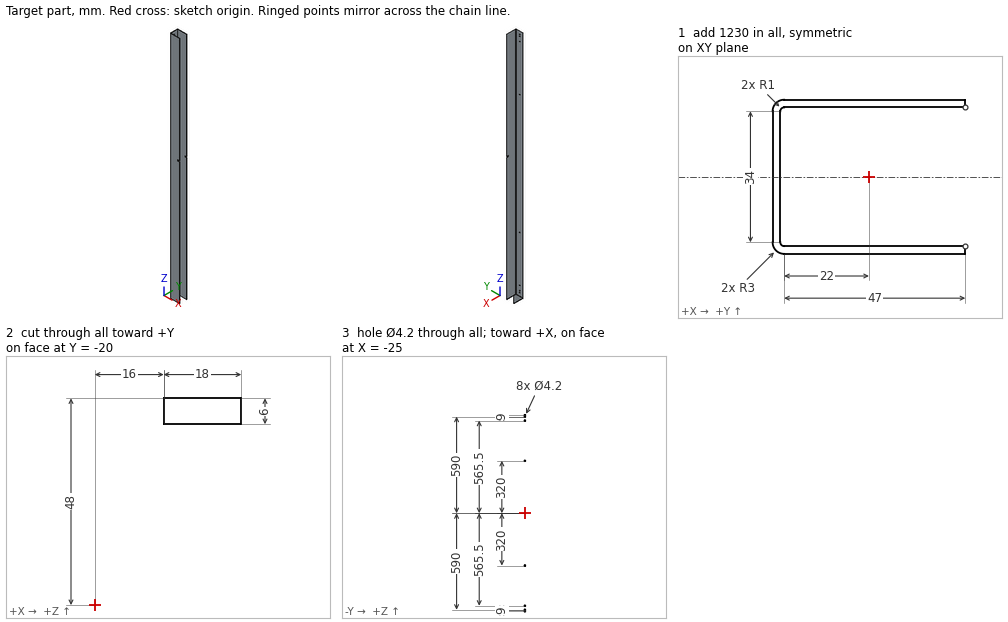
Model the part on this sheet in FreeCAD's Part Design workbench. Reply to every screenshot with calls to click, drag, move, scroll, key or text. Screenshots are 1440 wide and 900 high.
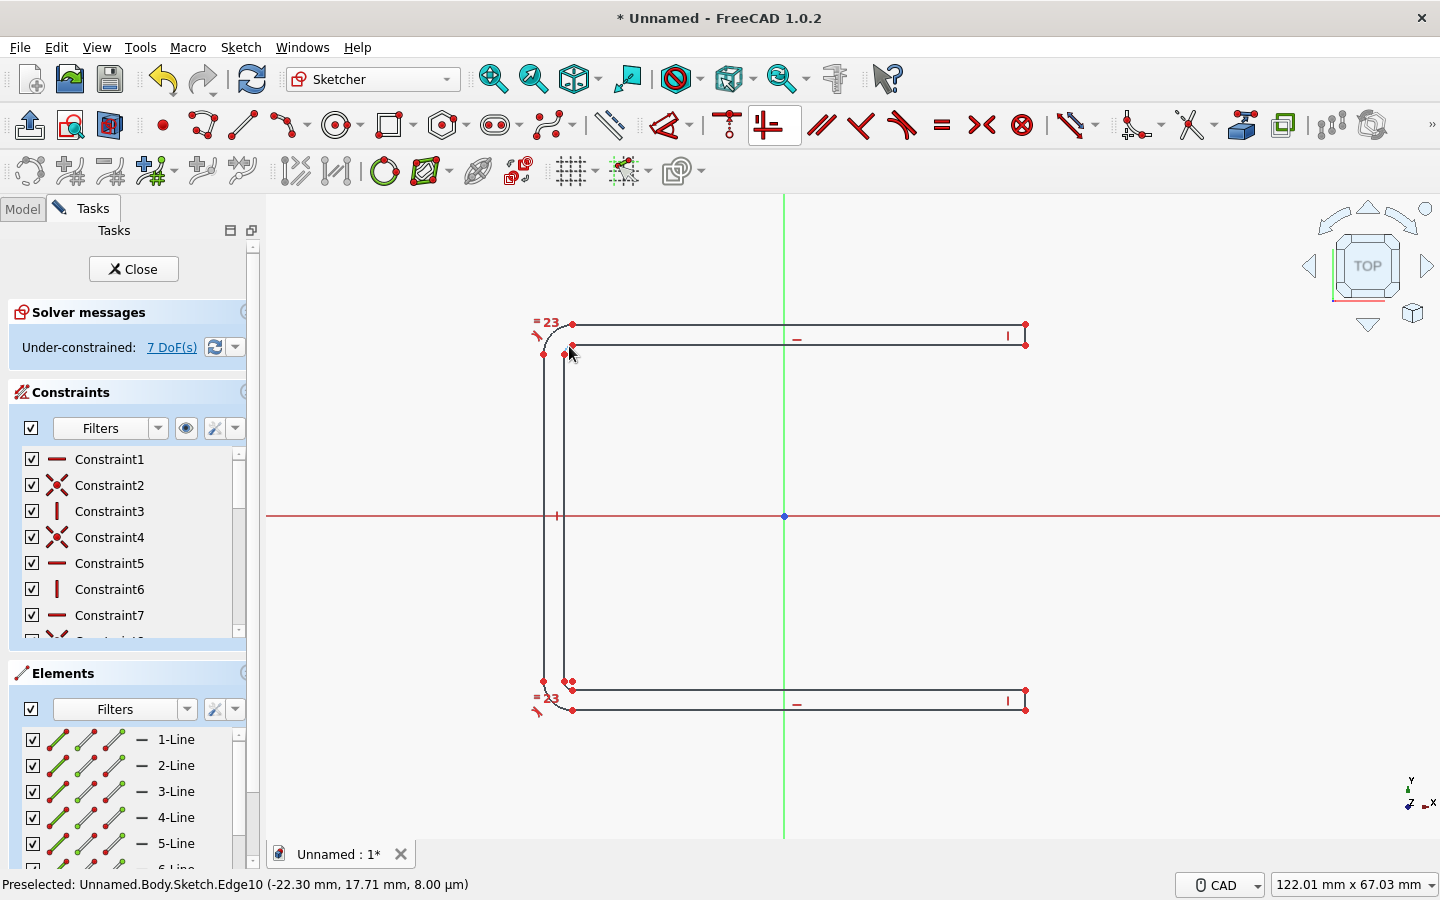
click(1025, 690)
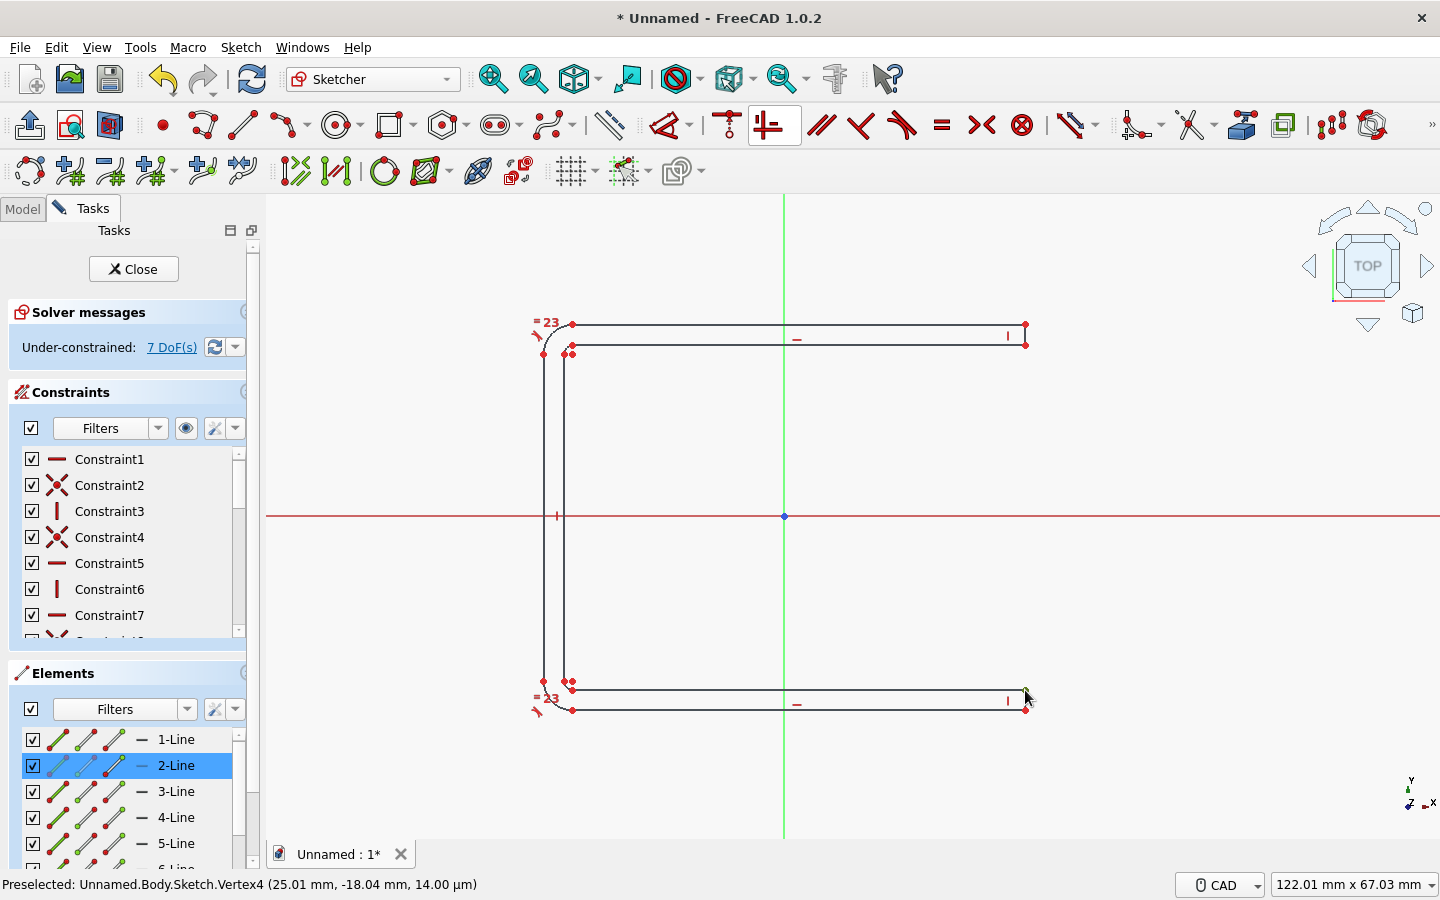
click(1025, 345)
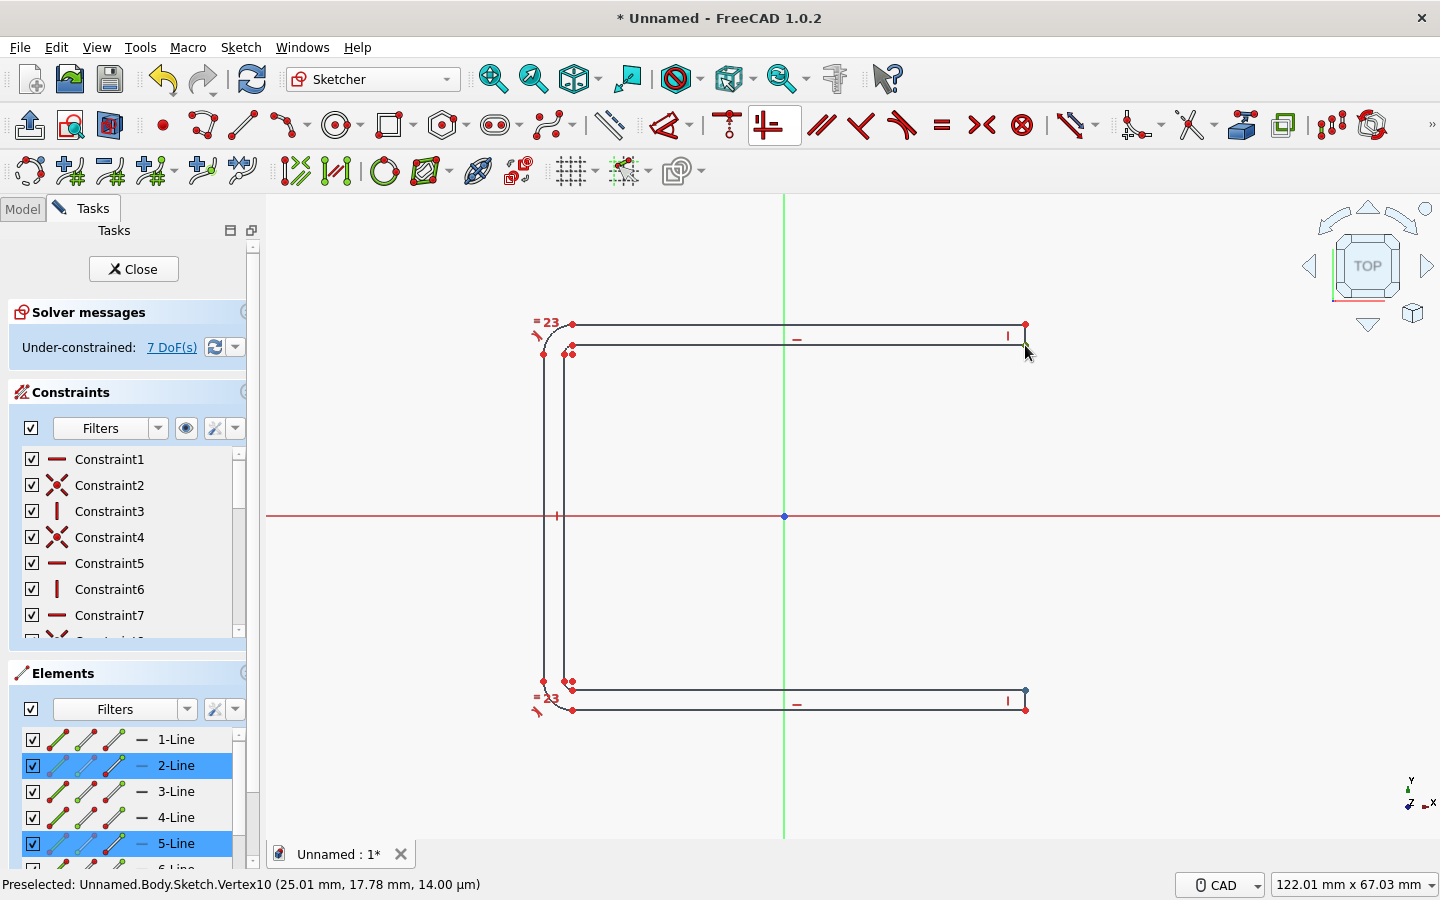
click(364, 516)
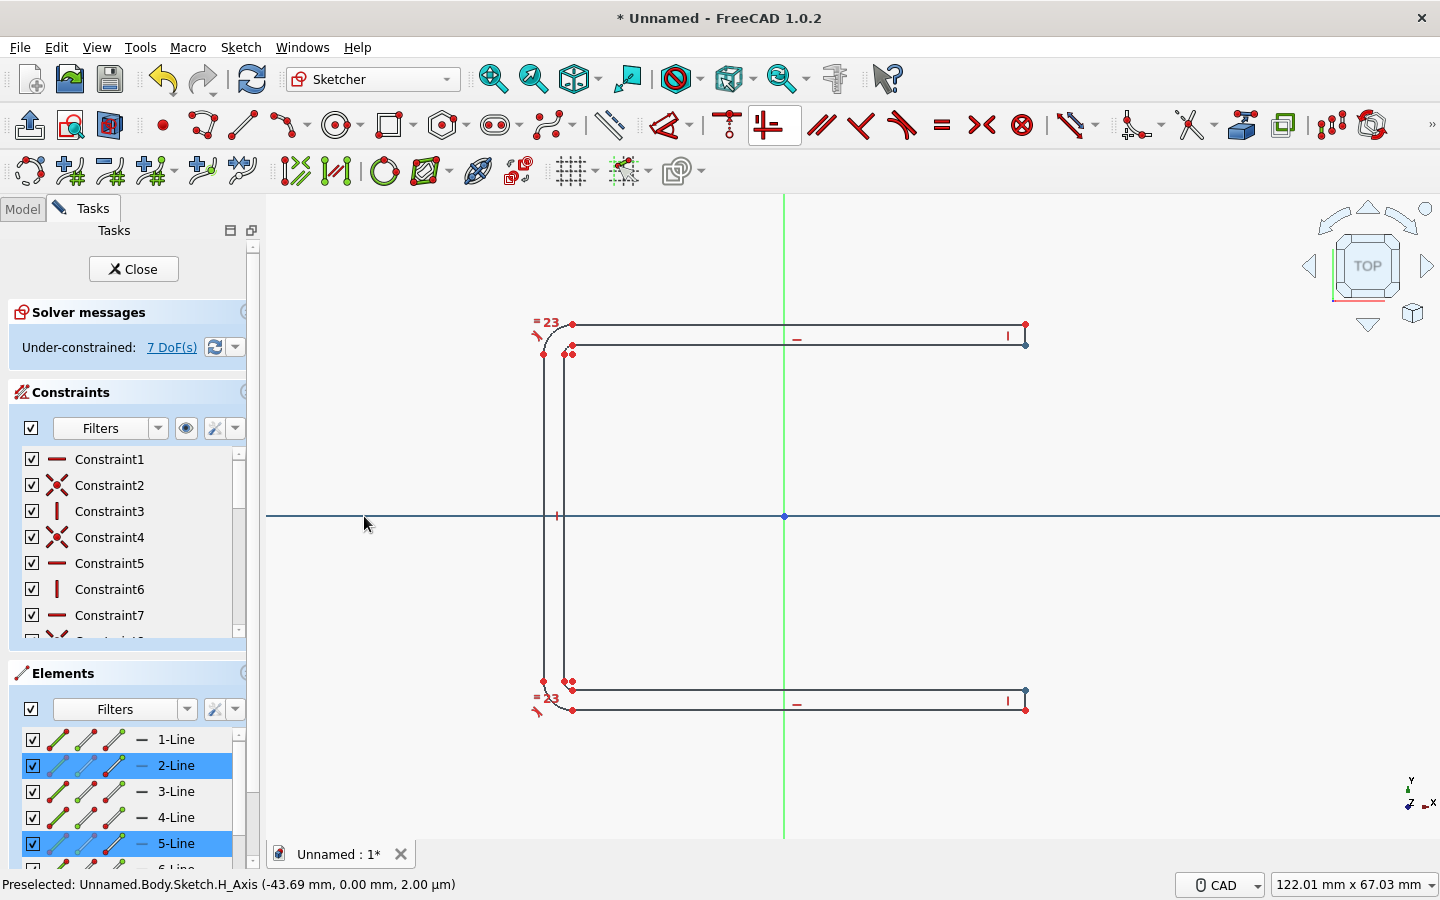
click(982, 126)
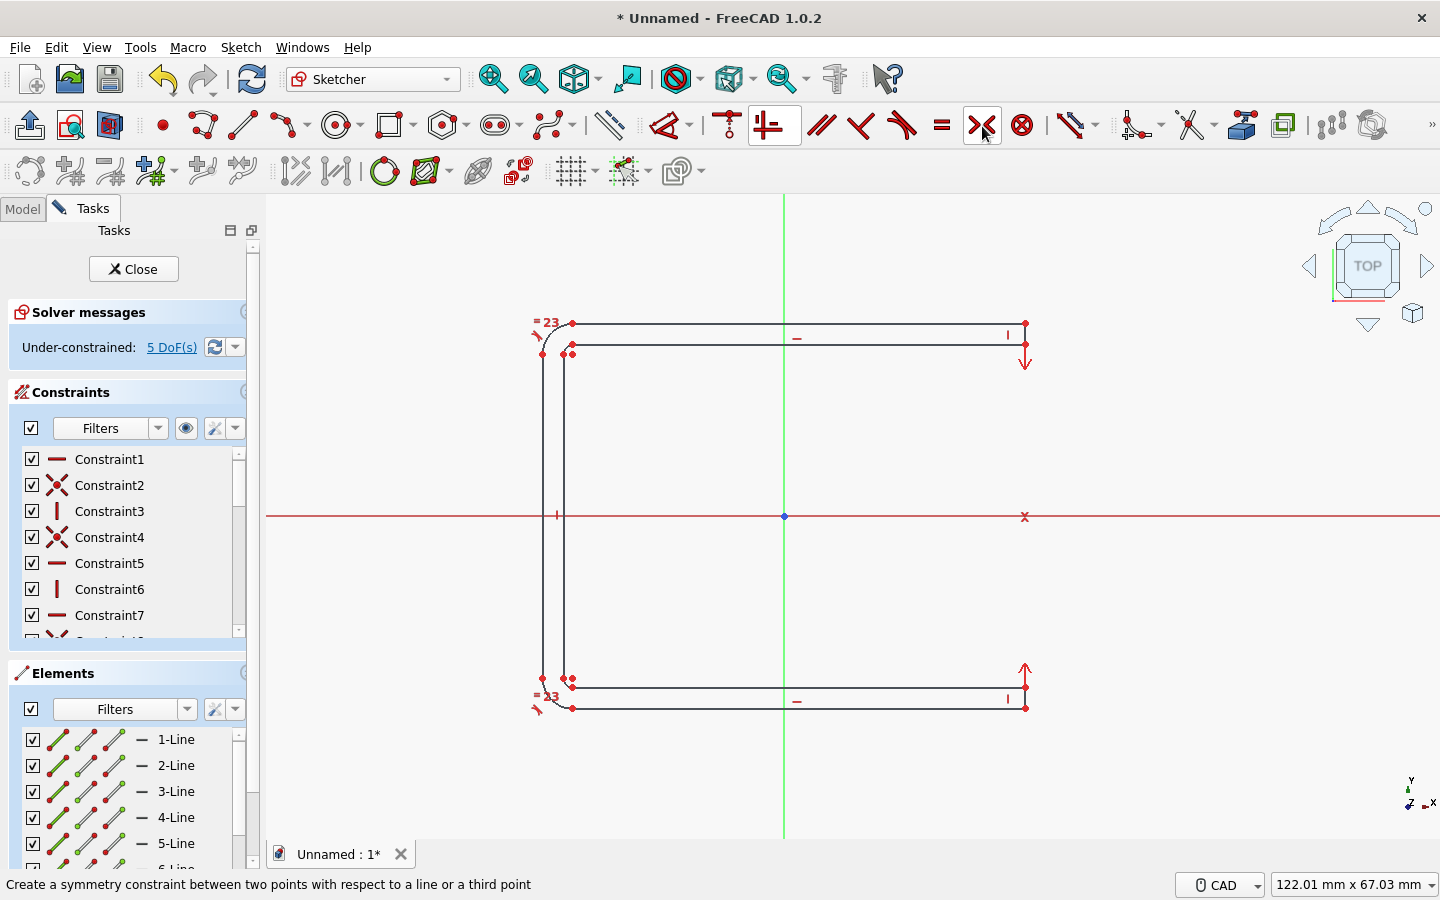
click(664, 126)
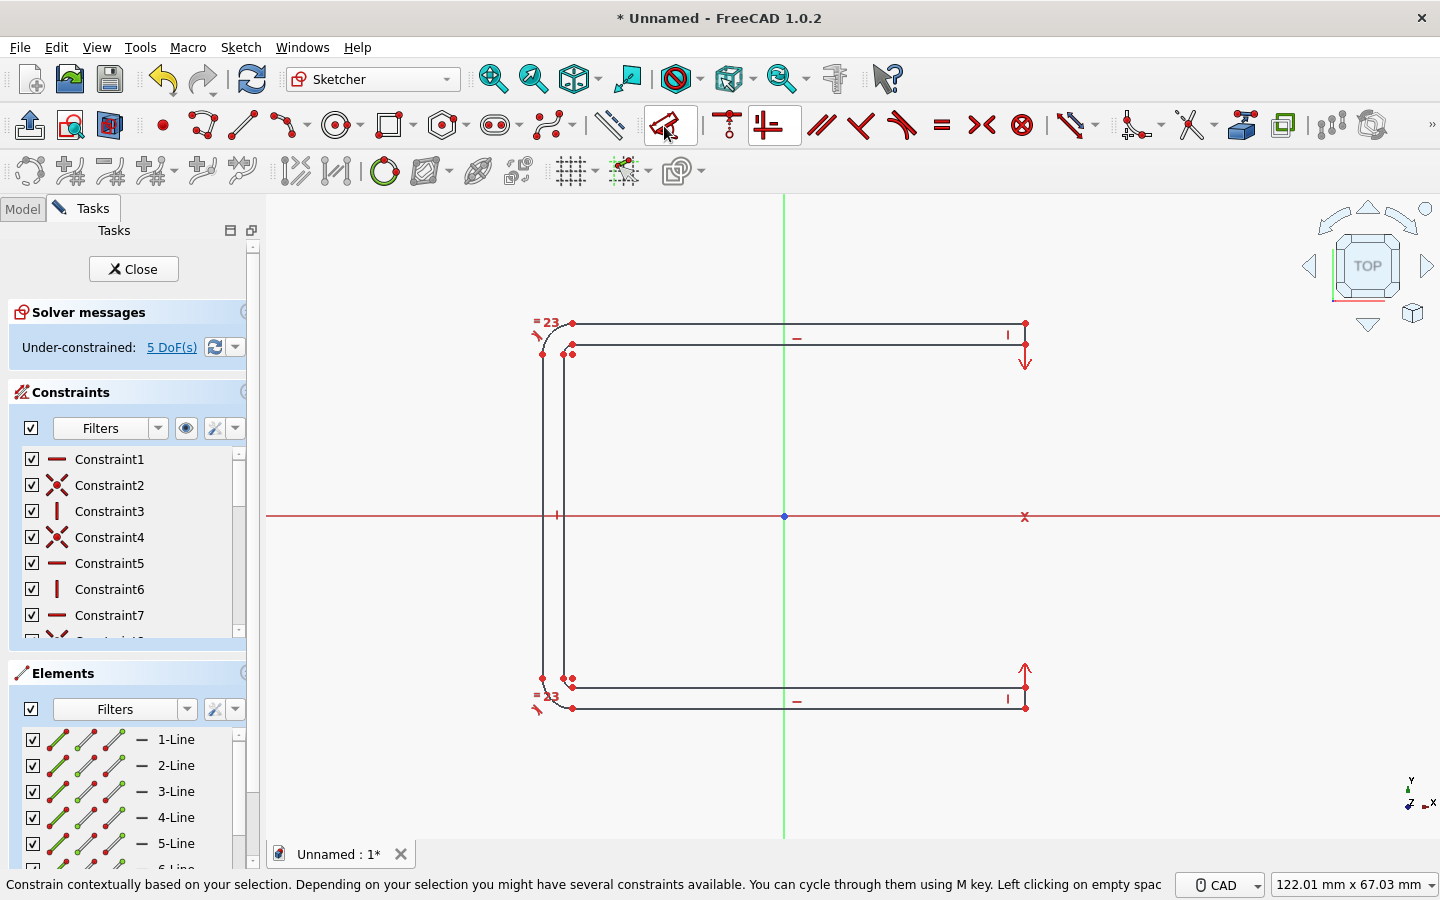
scroll(567, 685, up, 8)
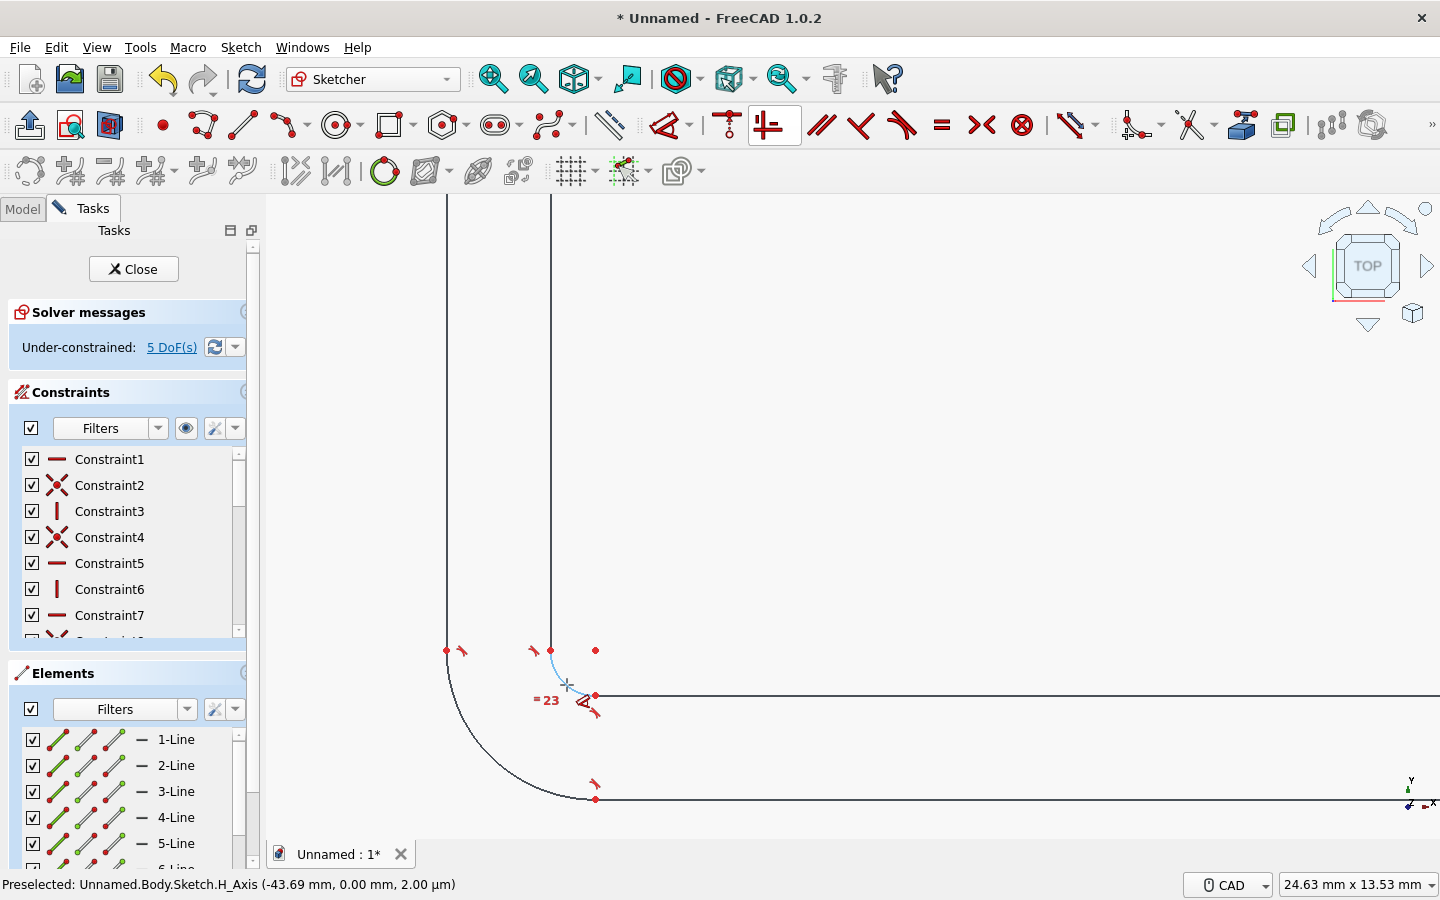
click(564, 683)
click(542, 706)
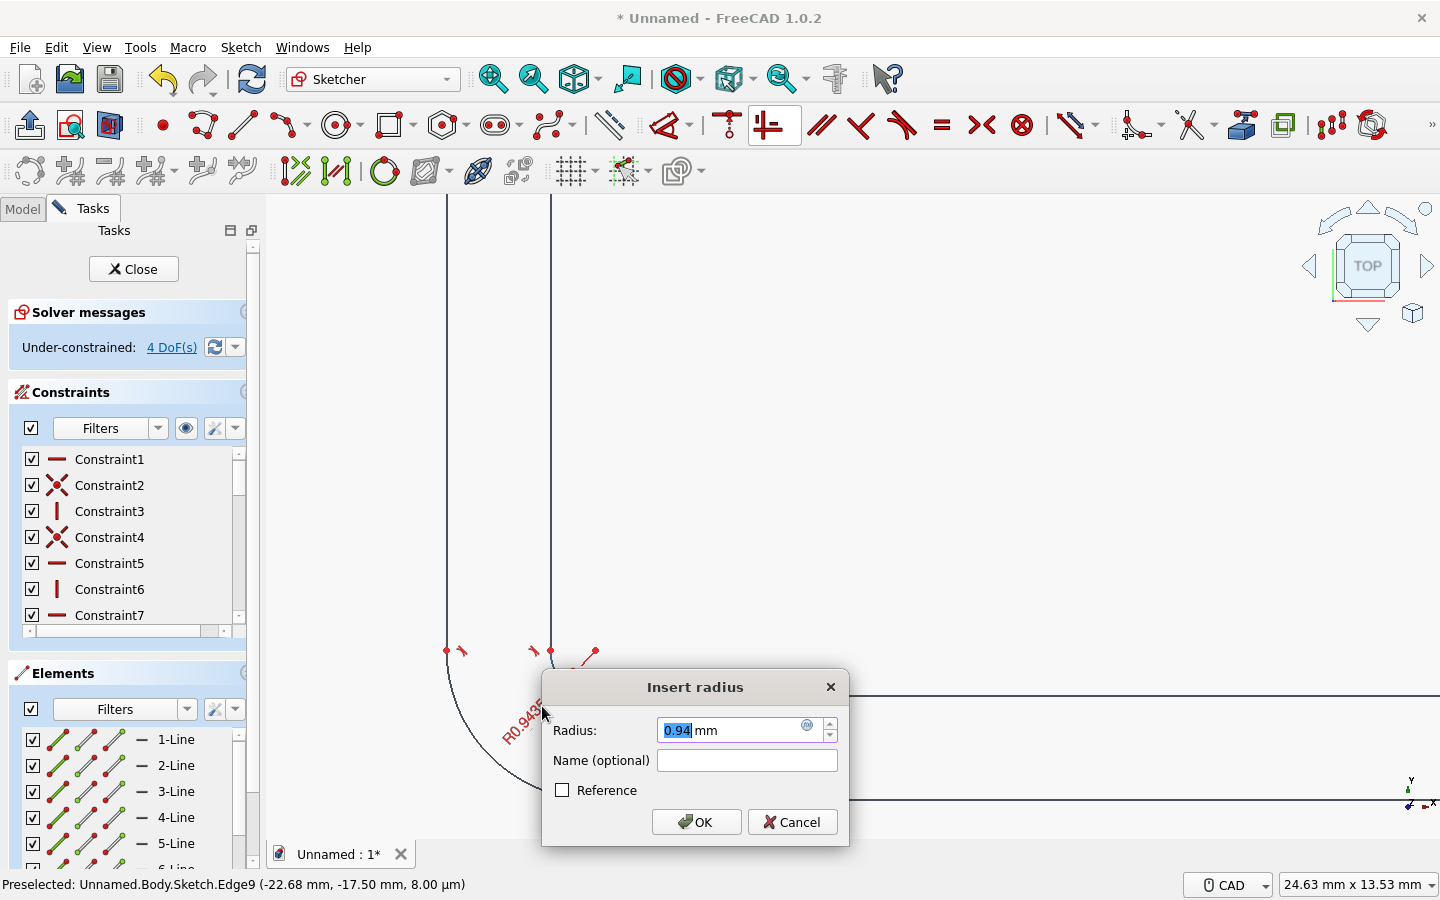
text(1)
key(Return)